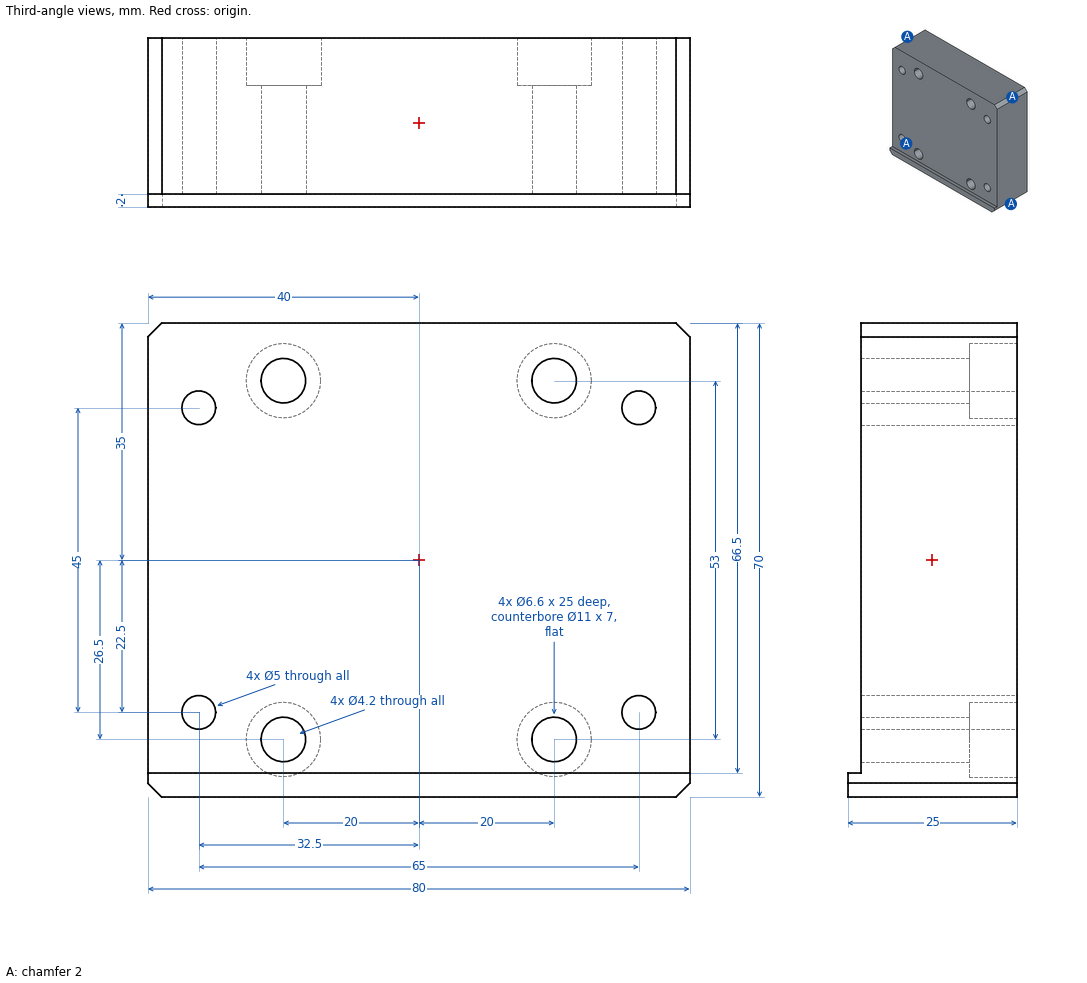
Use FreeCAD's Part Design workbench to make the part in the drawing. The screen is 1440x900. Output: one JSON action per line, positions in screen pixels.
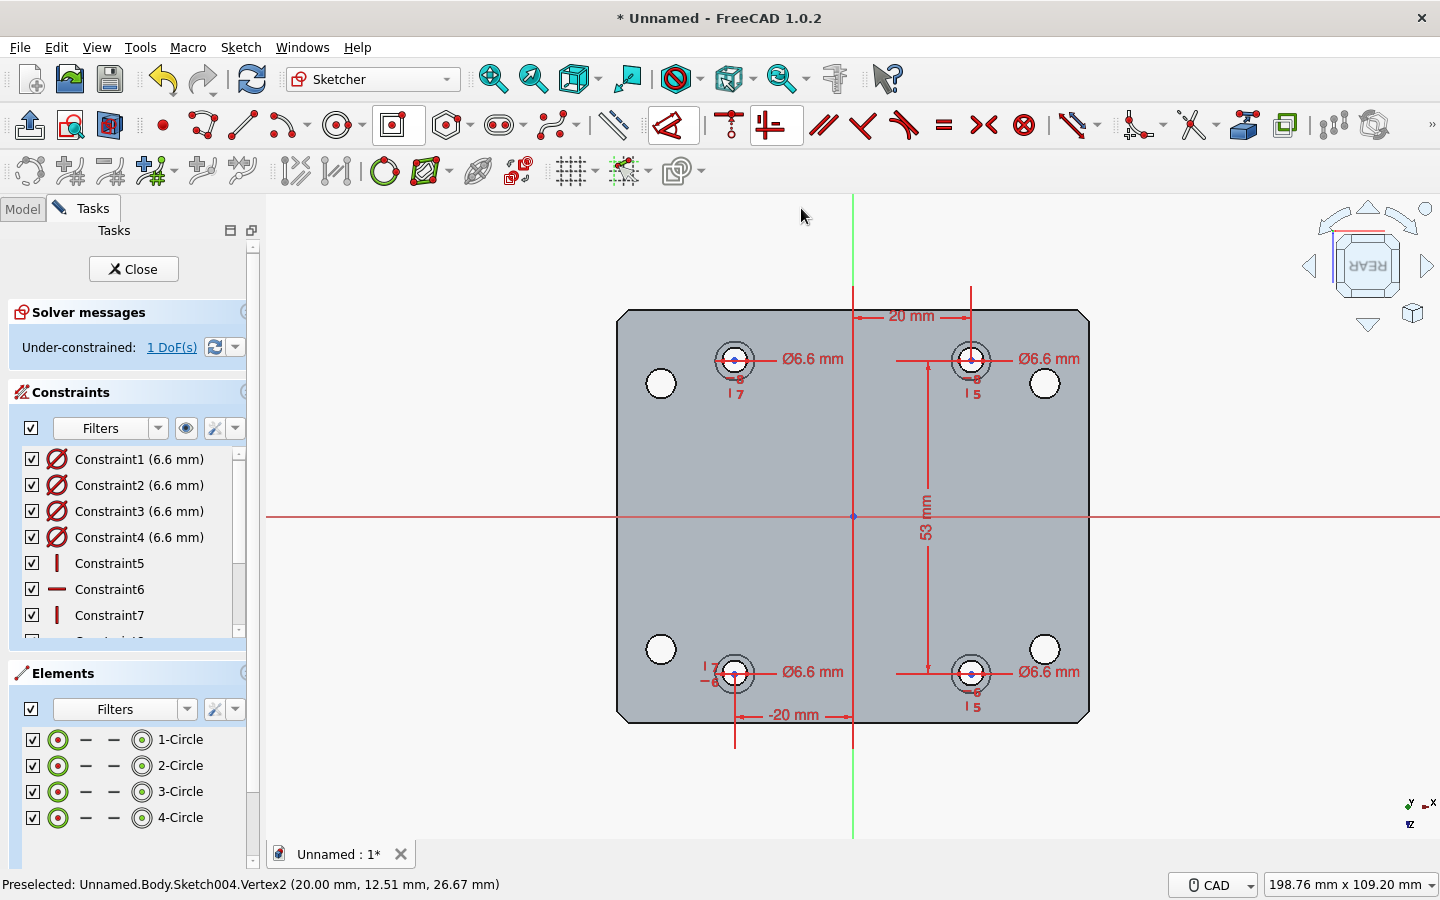
{"action": "left_click", "coordinate": [971, 361]}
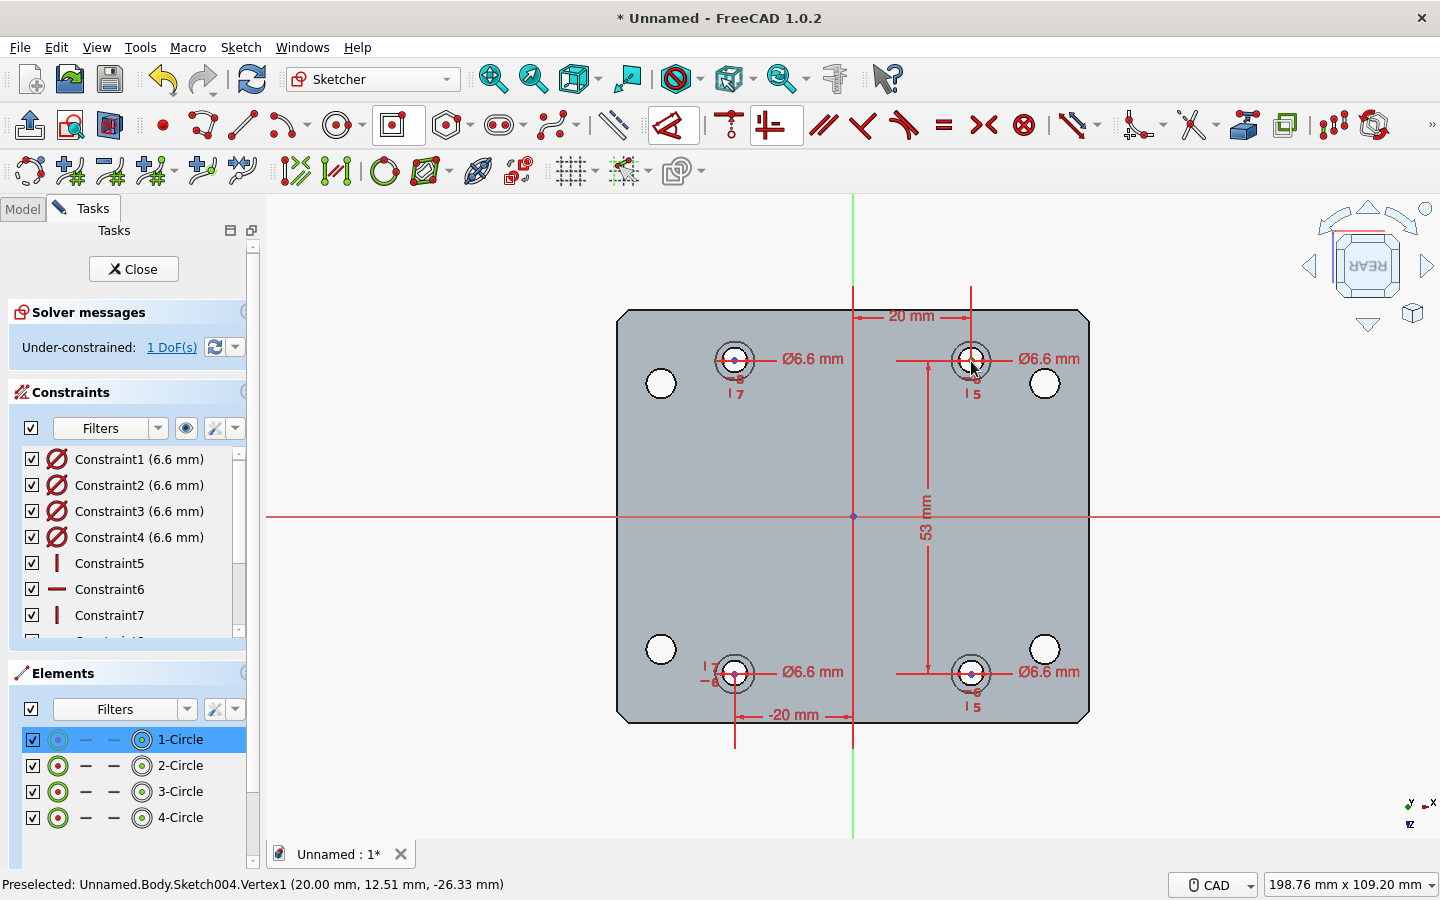
{"action": "left_click", "coordinate": [694, 126]}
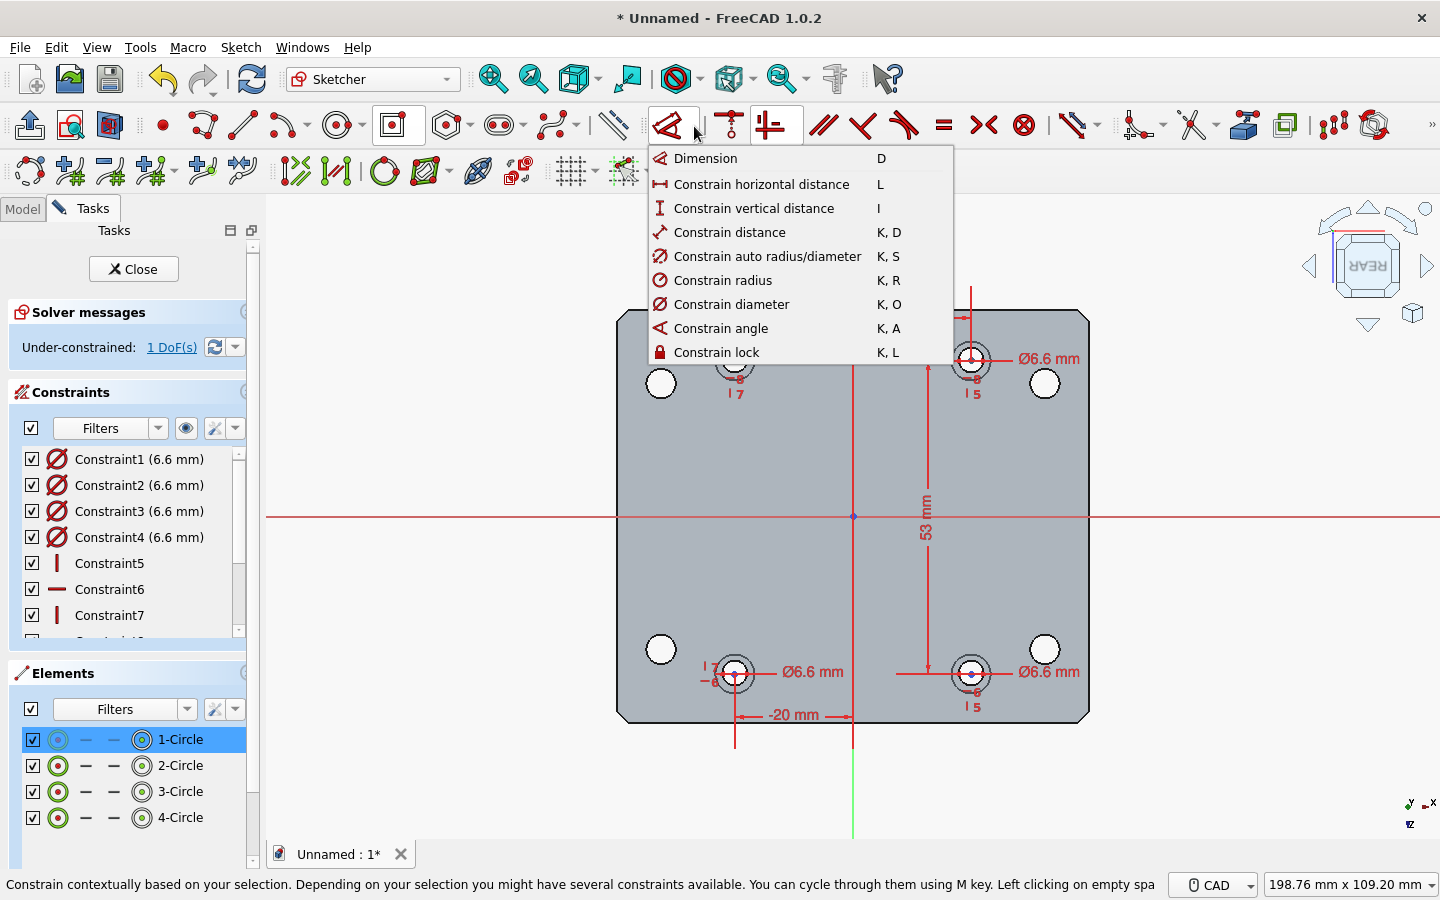
{"action": "left_click", "coordinate": [801, 208]}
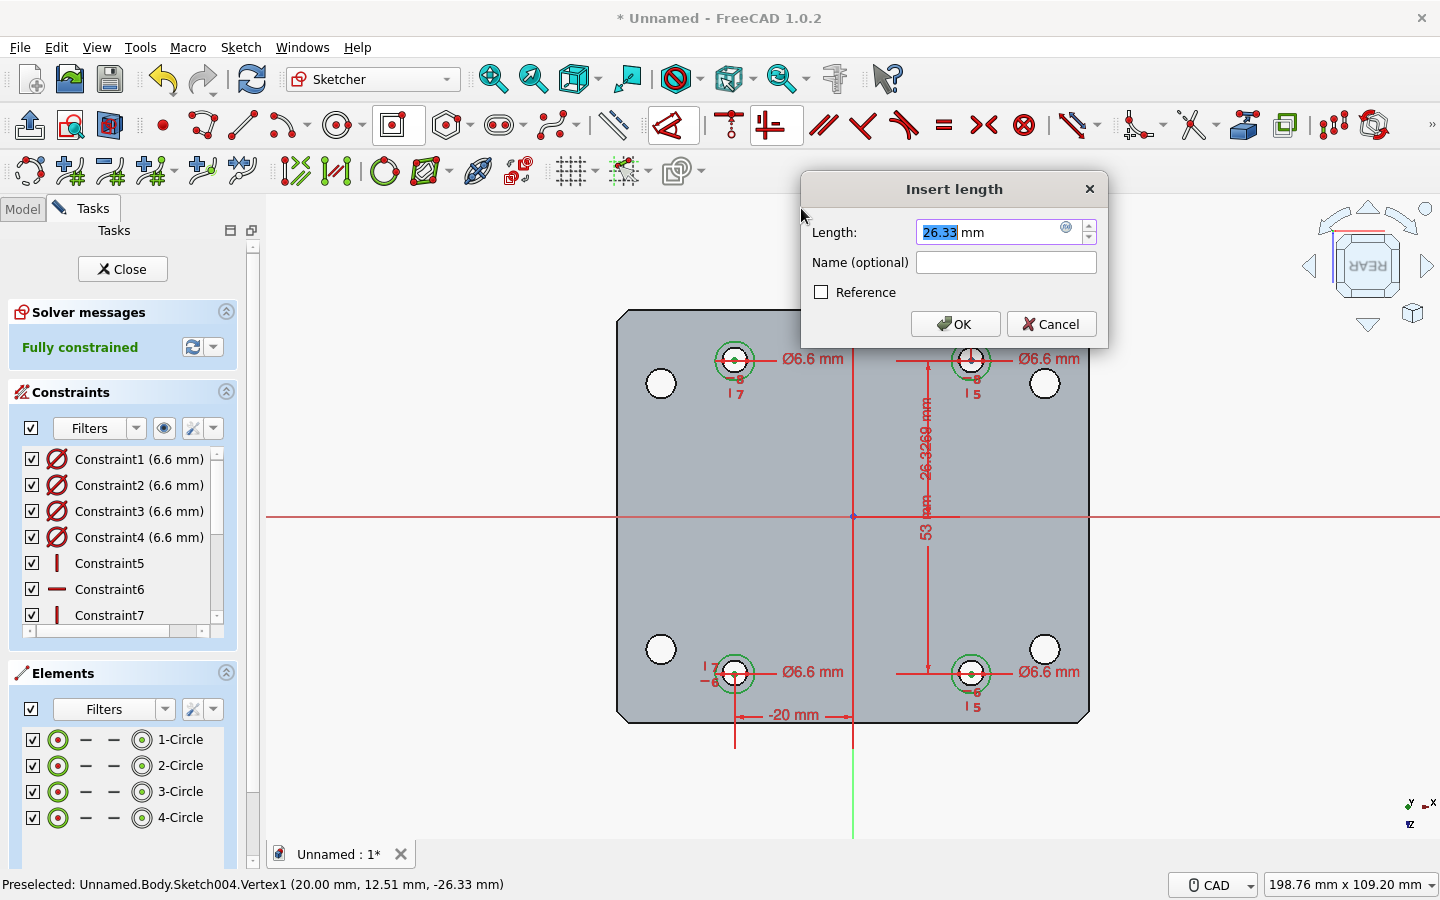
{"action": "type", "text": "26.5"}
{"action": "key", "text": "Return"}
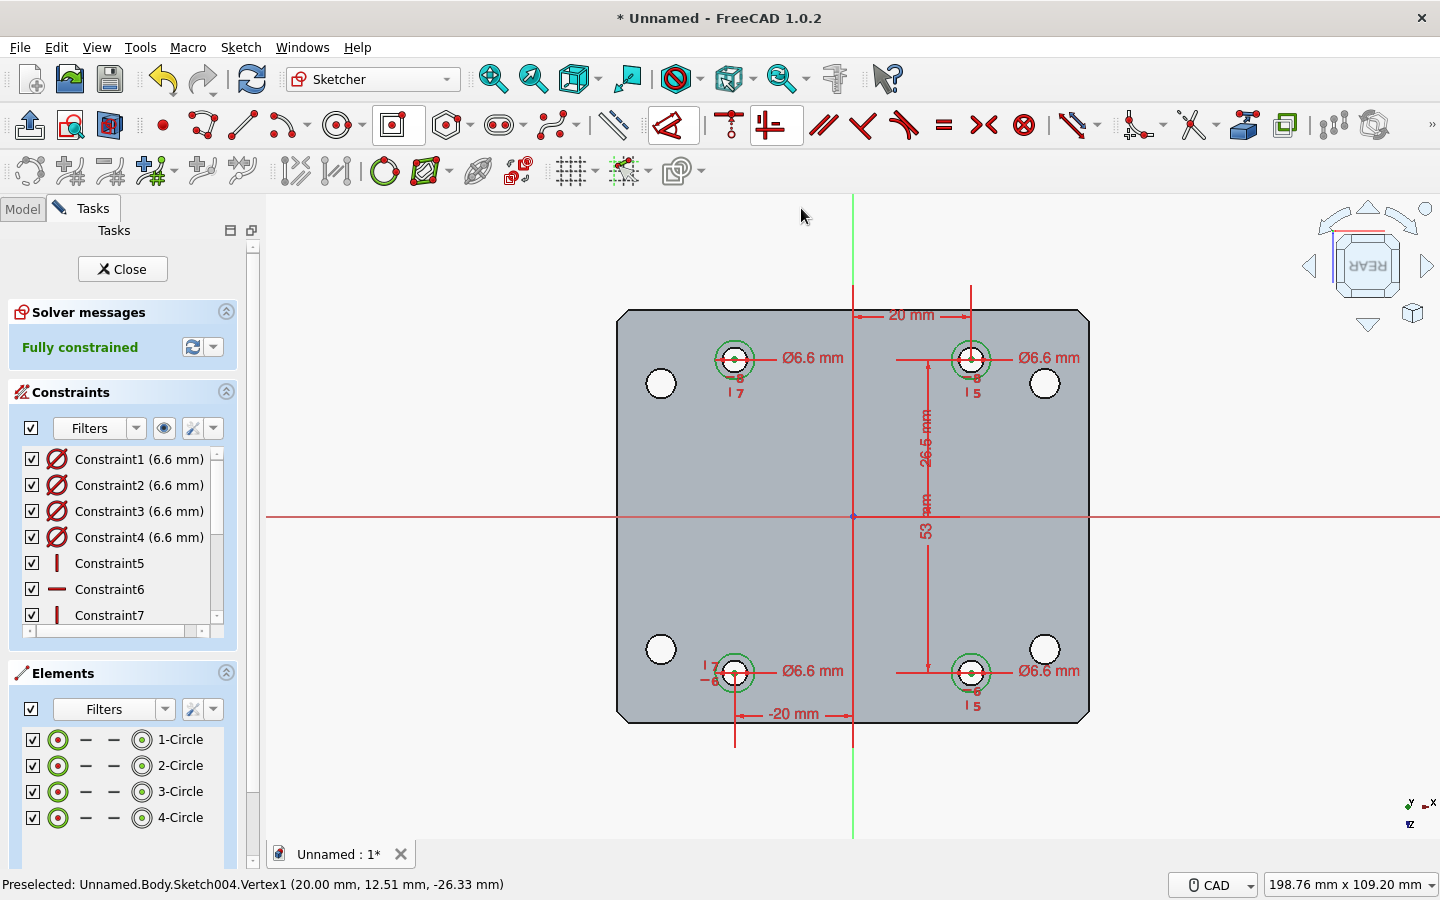
{"action": "left_click", "coordinate": [123, 269]}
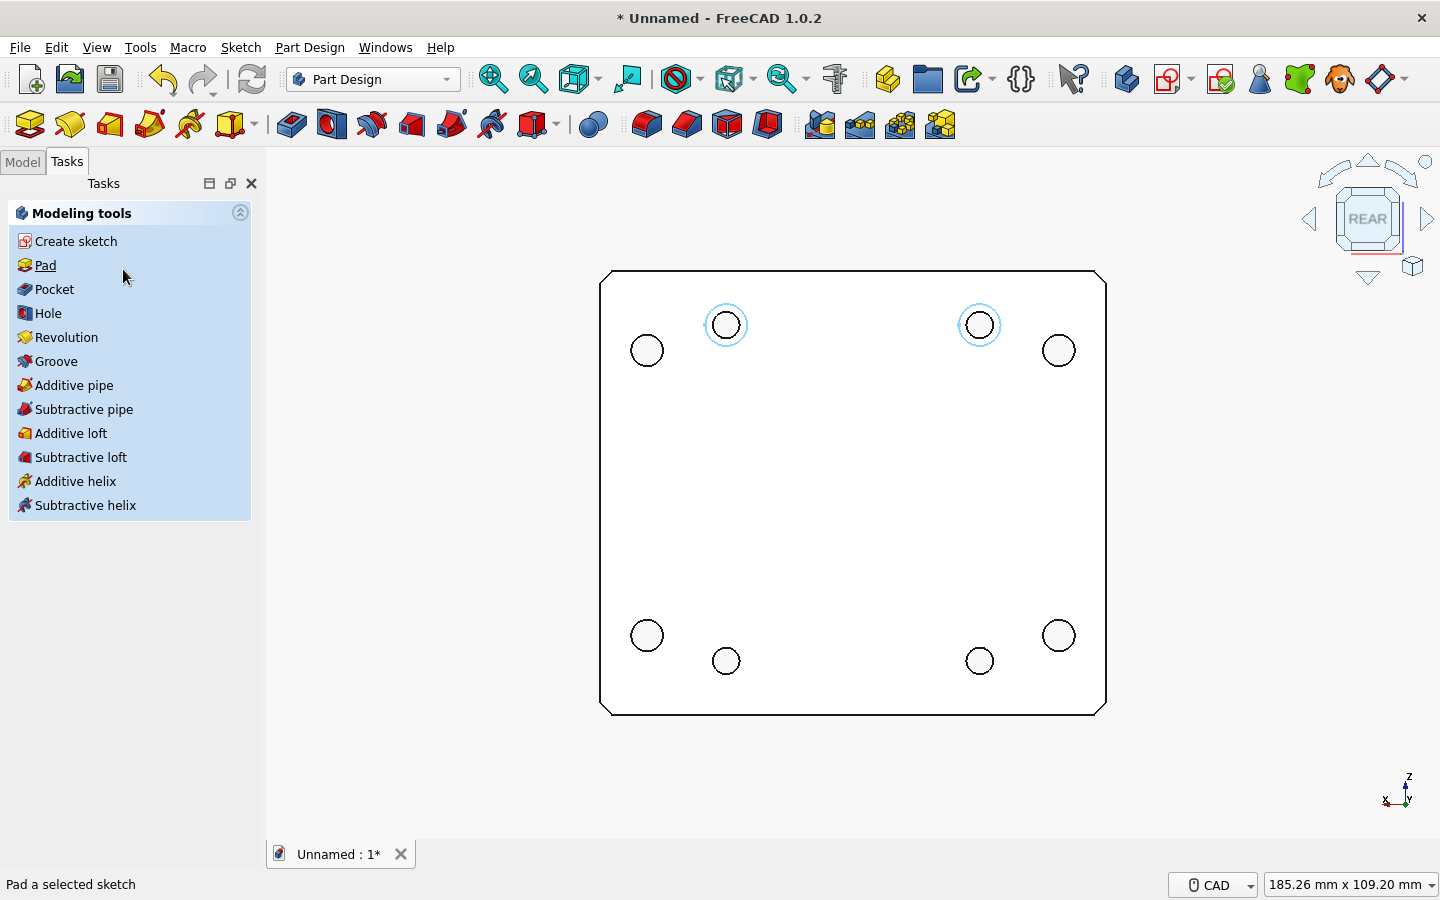
{"action": "left_click", "coordinate": [332, 124]}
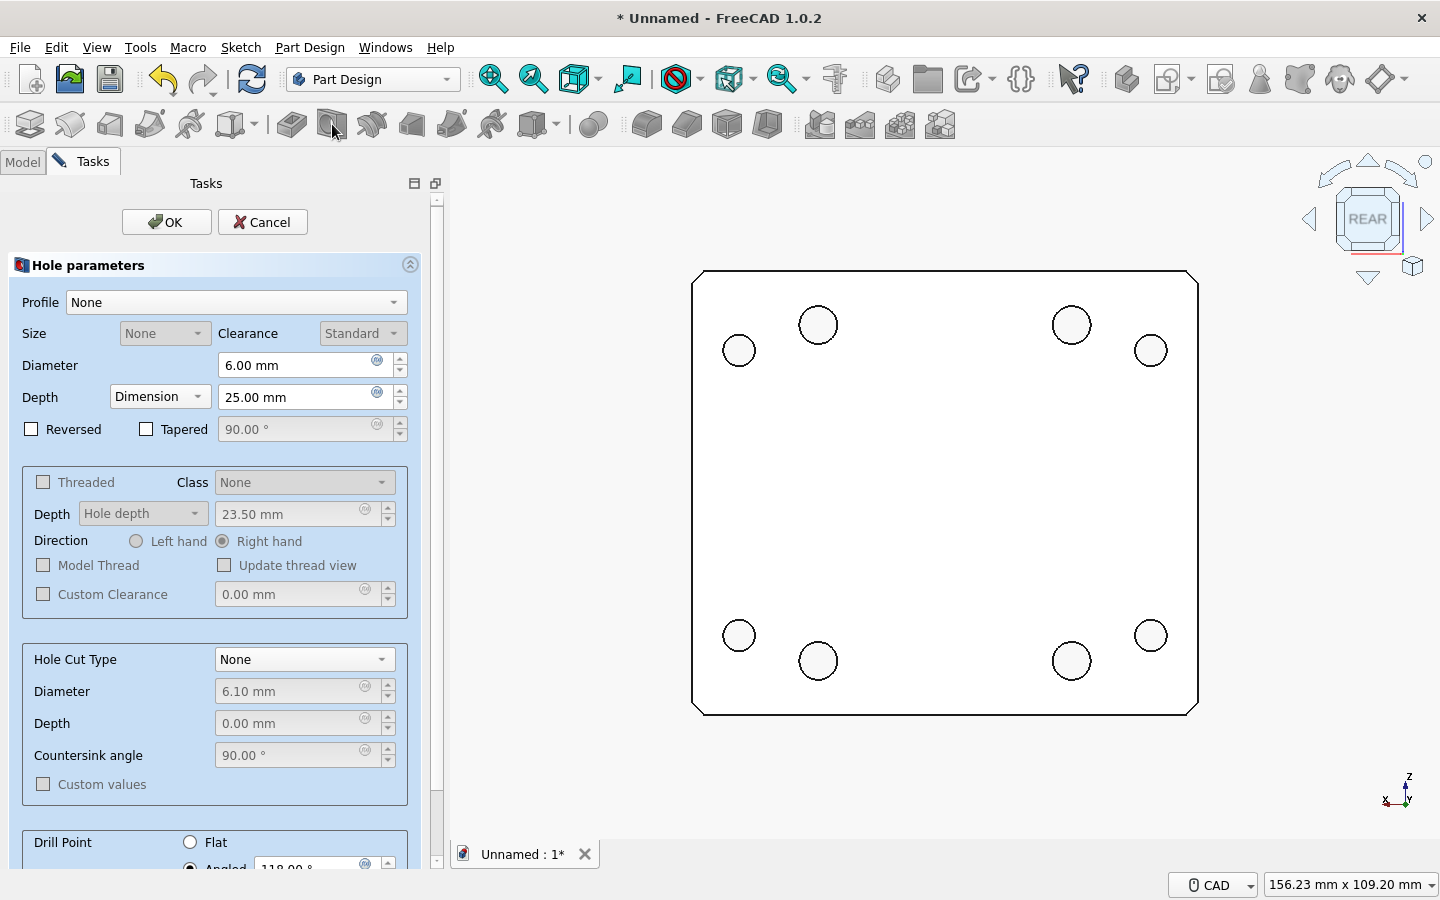
{"action": "triple_click", "coordinate": [305, 365]}